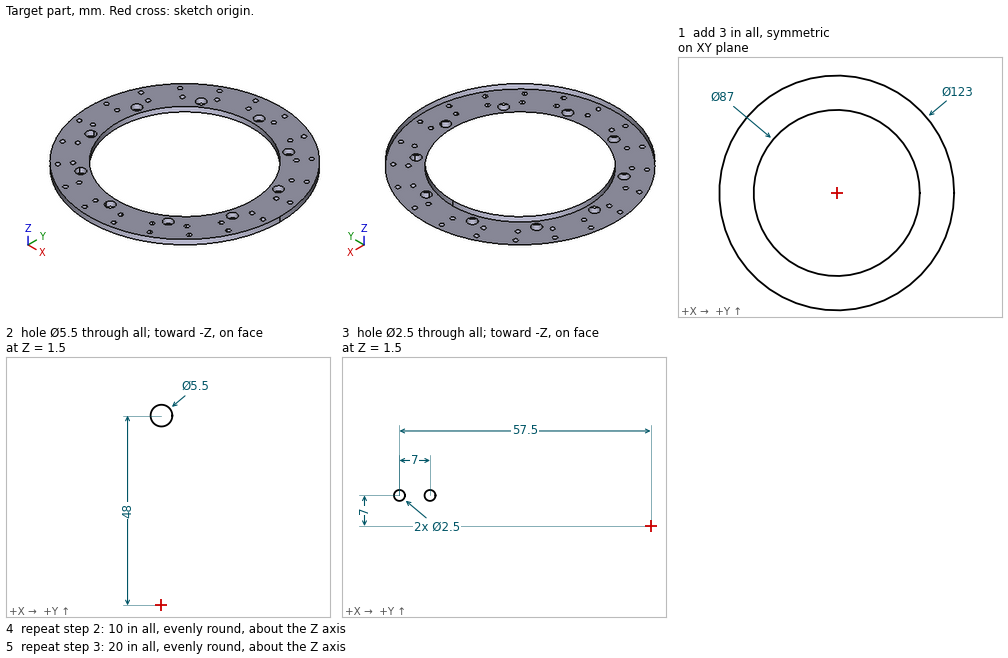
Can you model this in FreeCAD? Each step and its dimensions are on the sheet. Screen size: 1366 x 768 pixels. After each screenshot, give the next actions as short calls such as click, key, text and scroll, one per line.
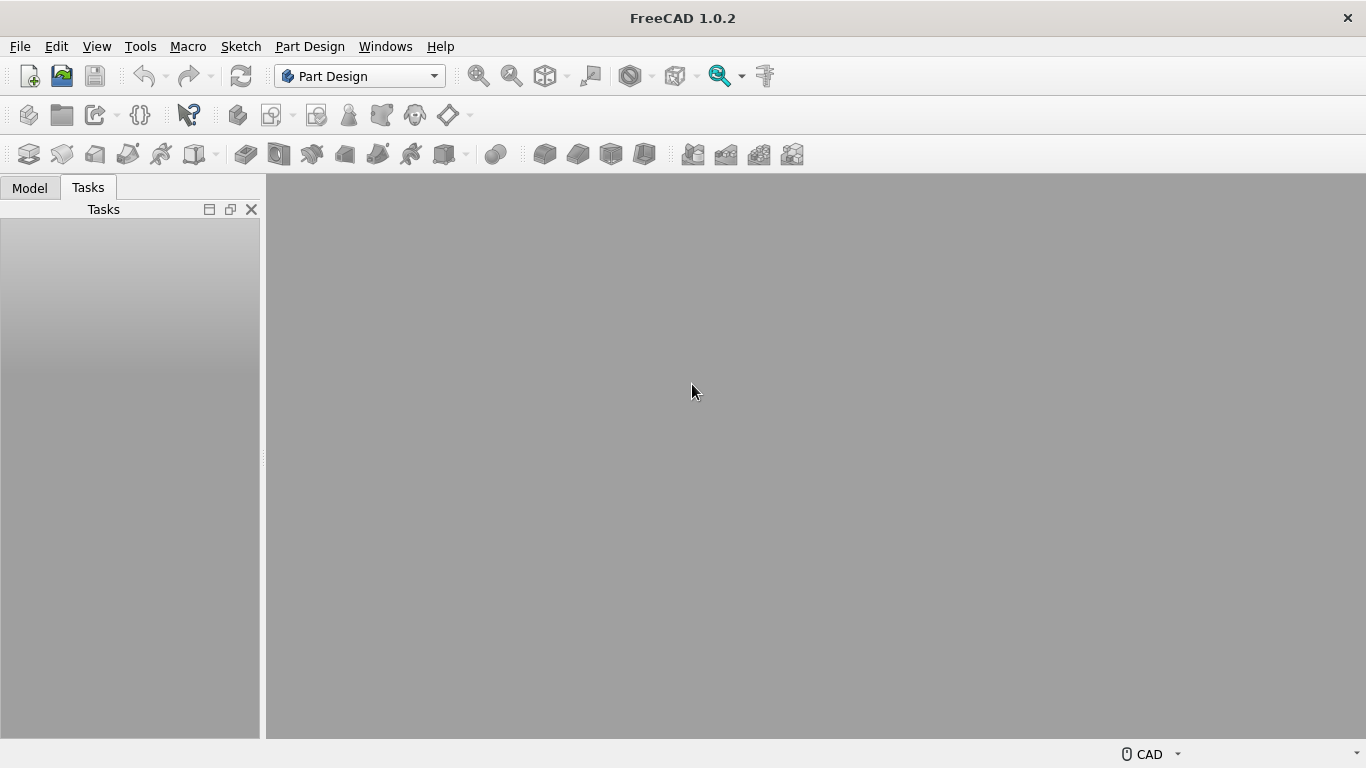
click(29, 76)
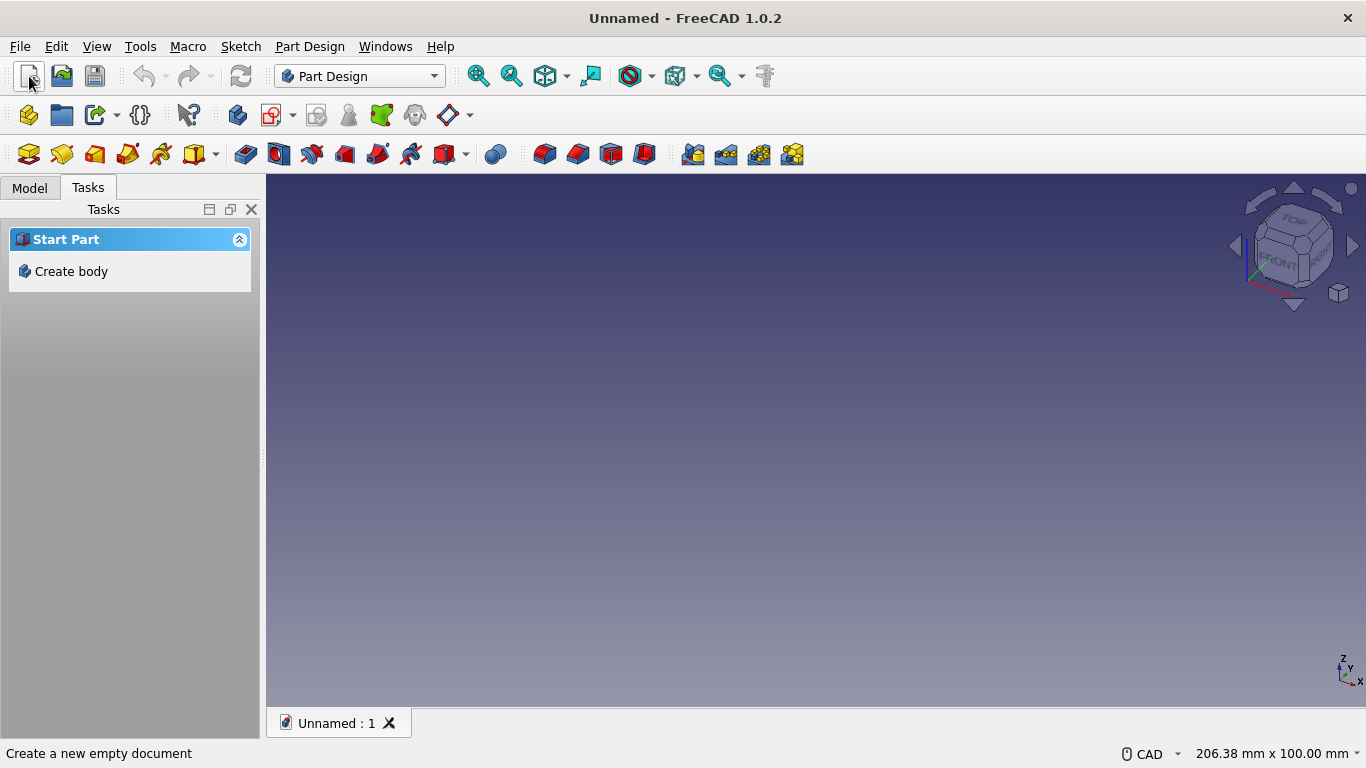
click(270, 116)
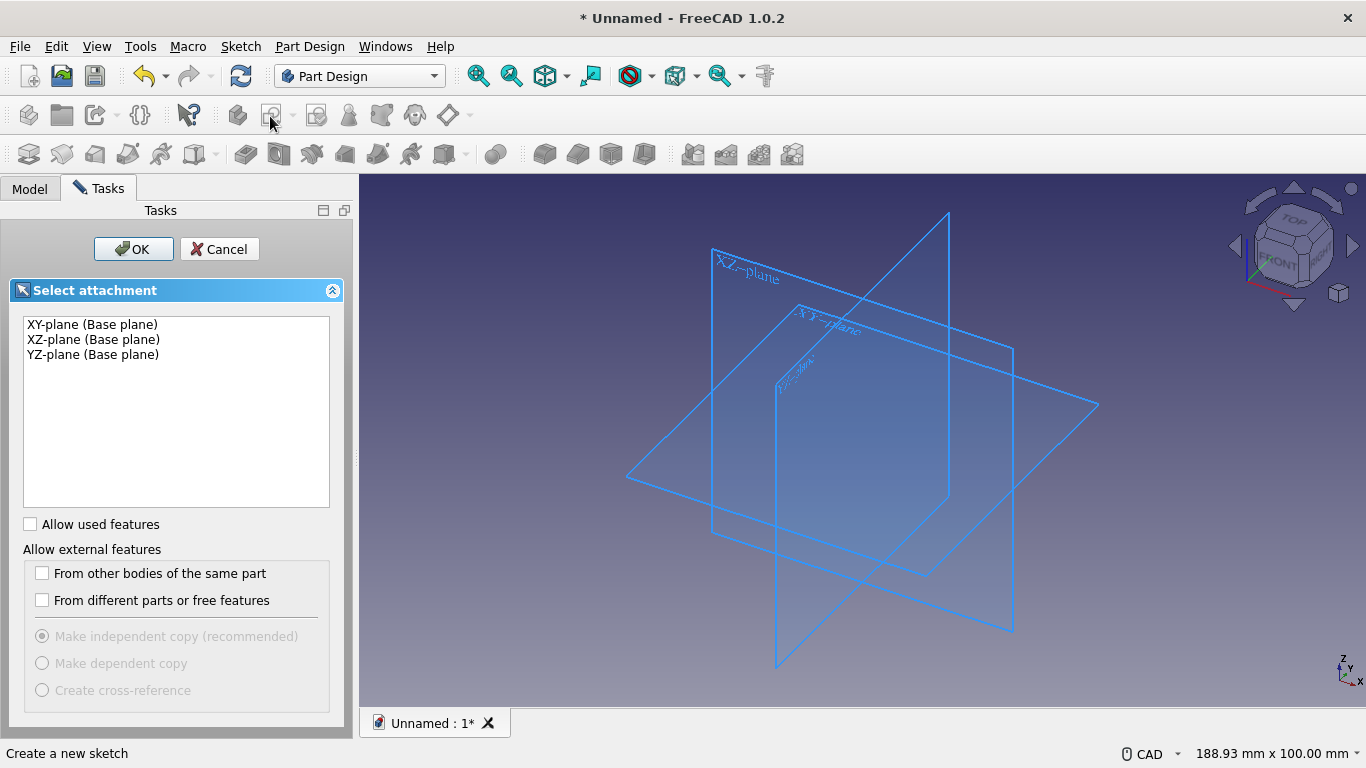
click(84, 324)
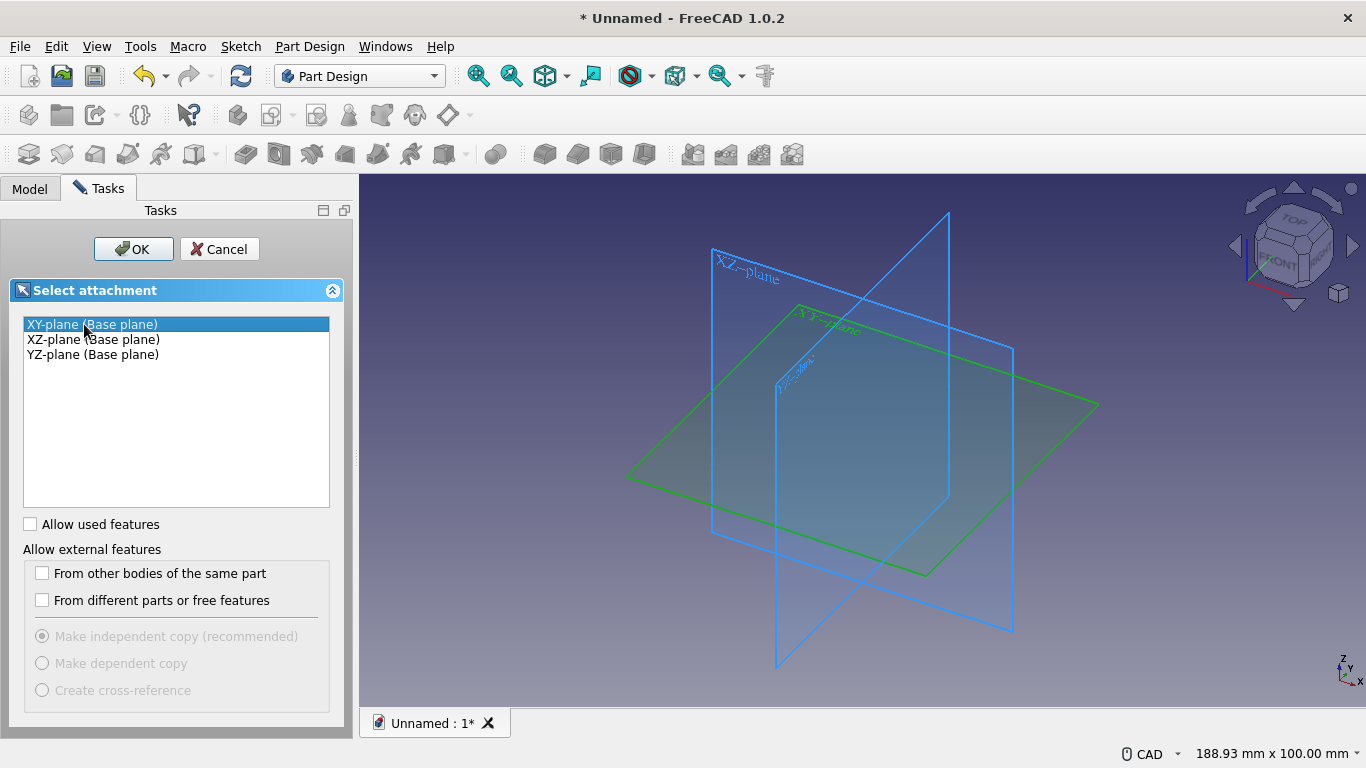
click(134, 249)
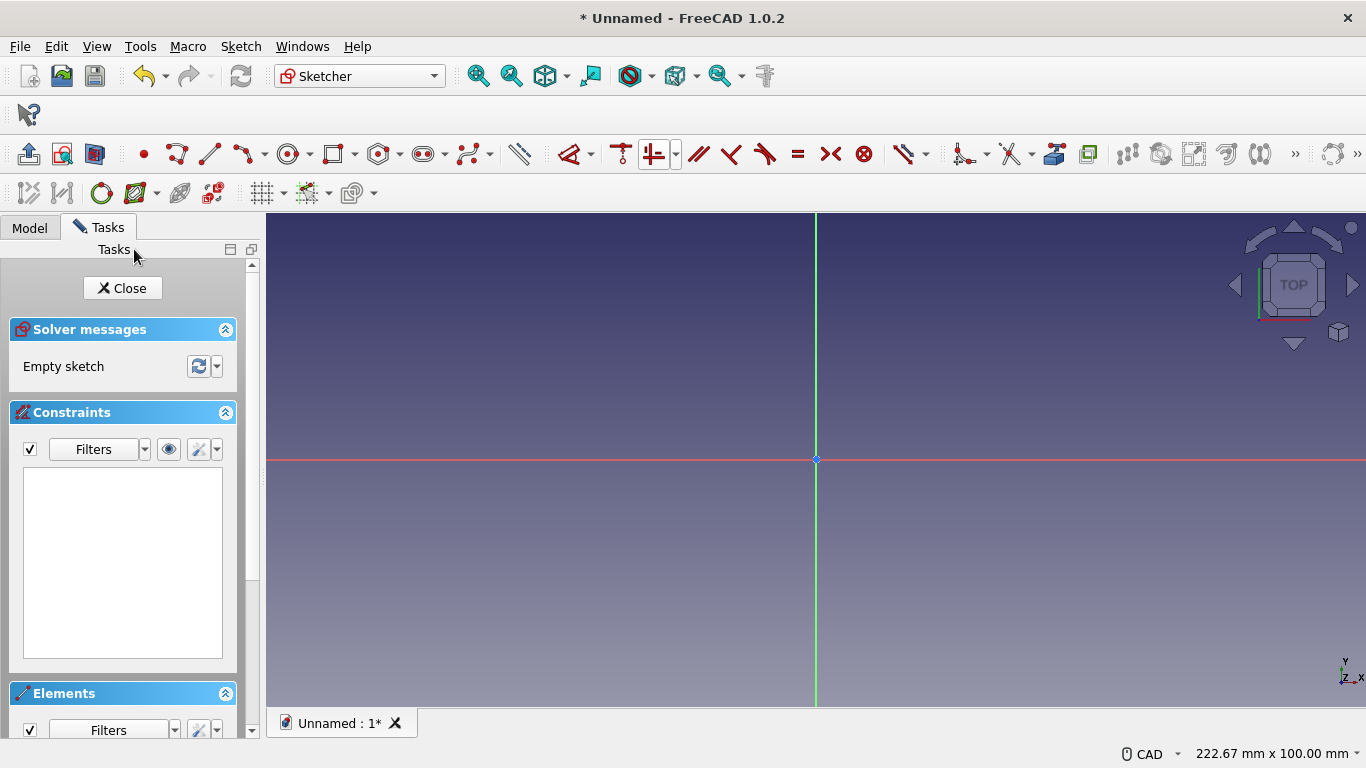
scroll(664, 460, down, 3)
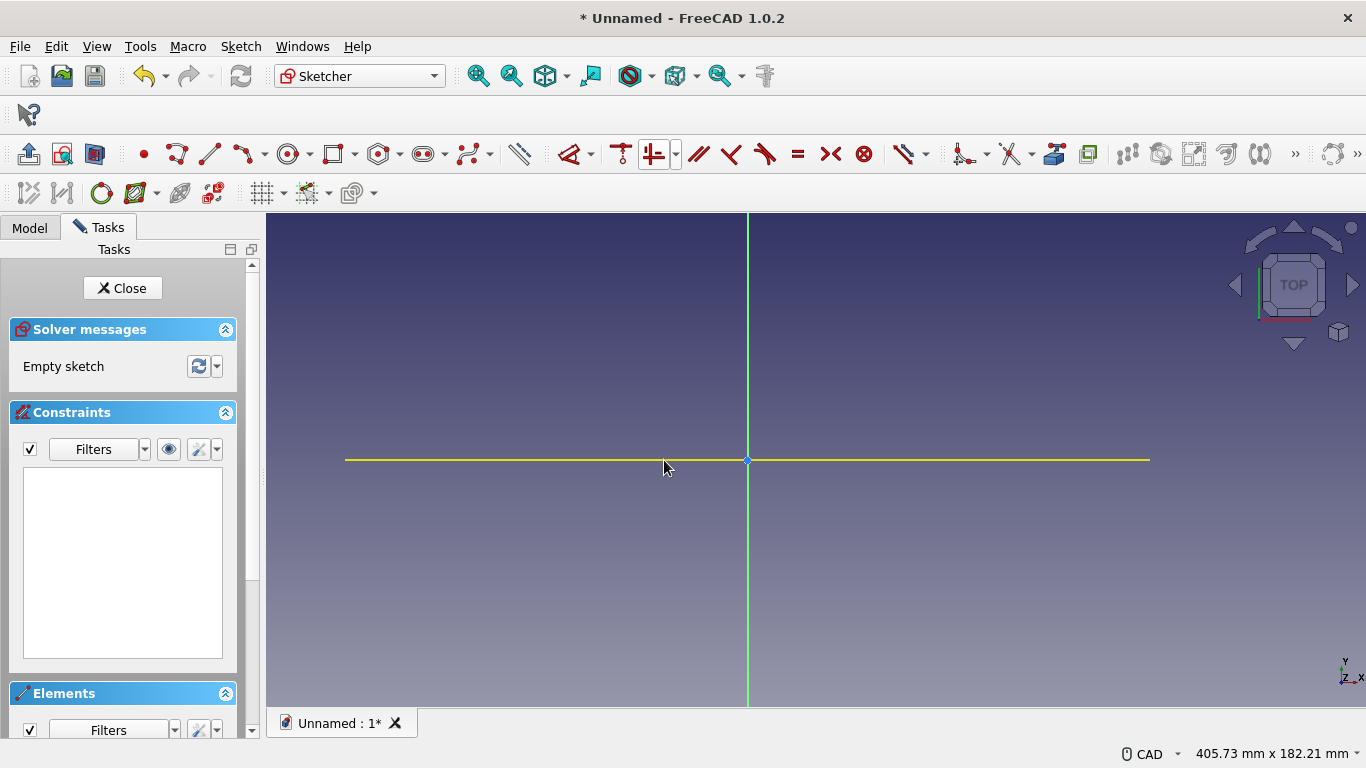
click(288, 154)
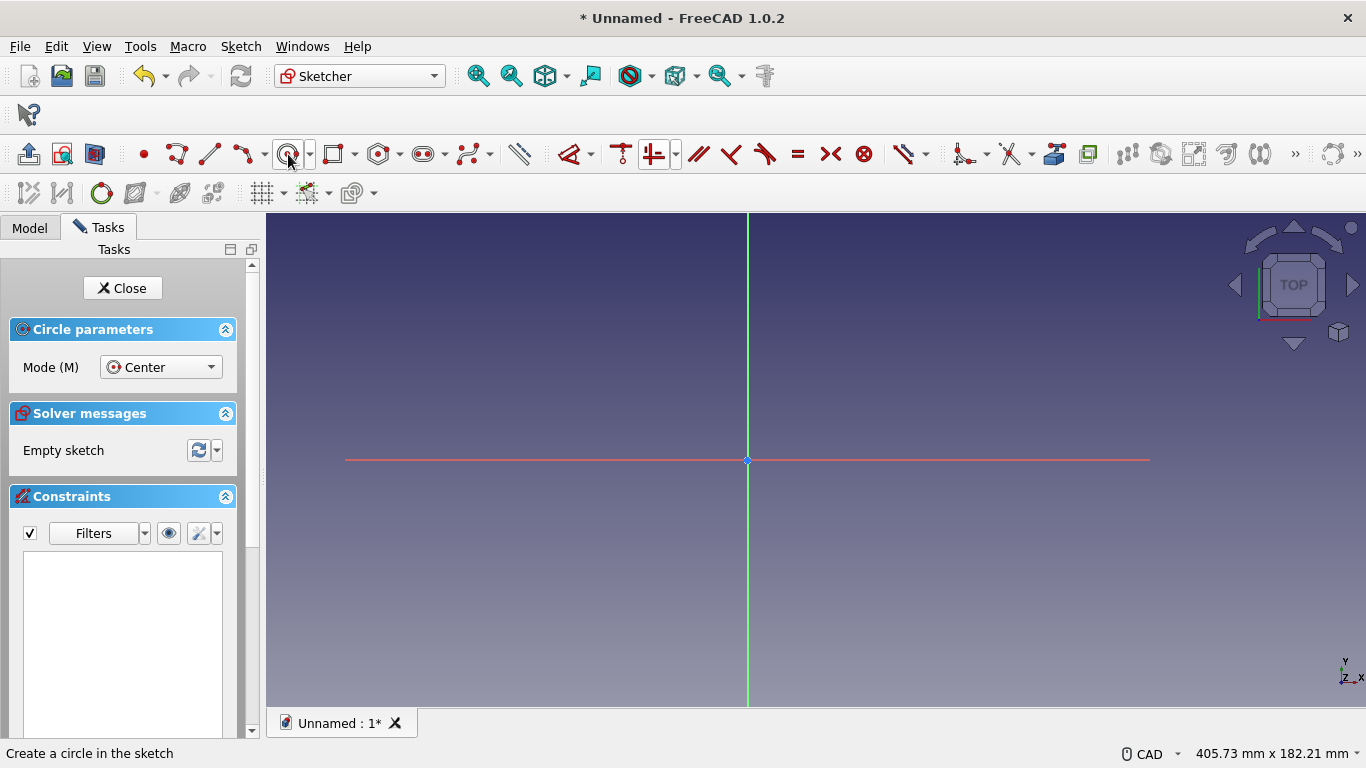
click(748, 460)
move(865, 342)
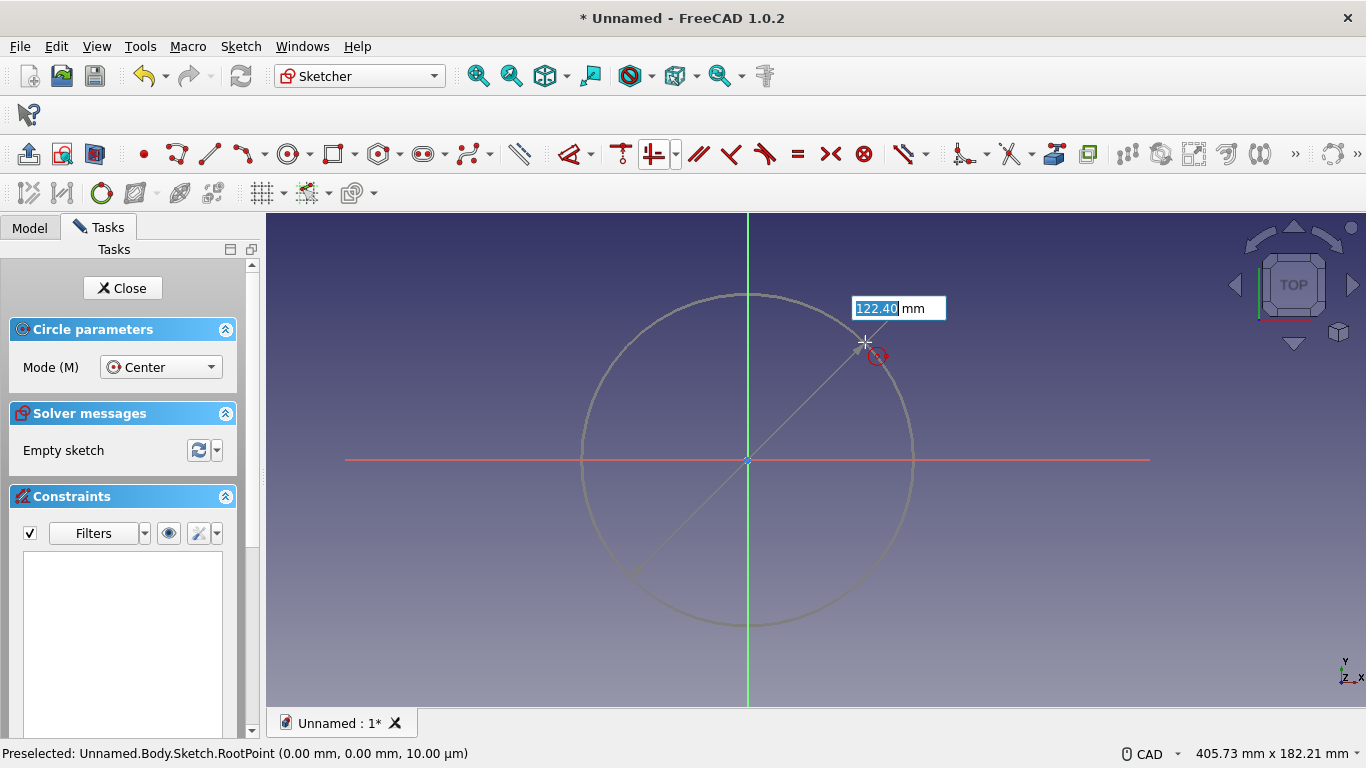
text(123)
key(Return)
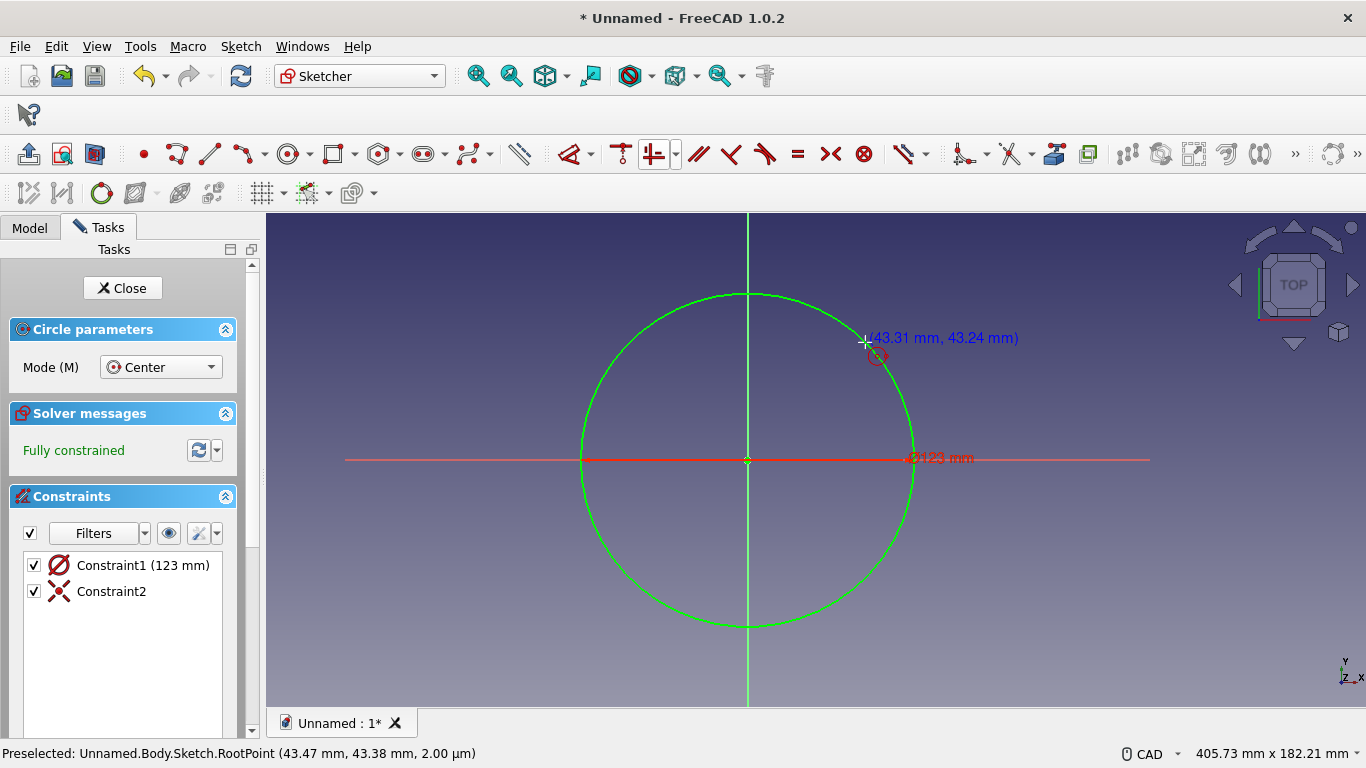
click(748, 460)
move(831, 377)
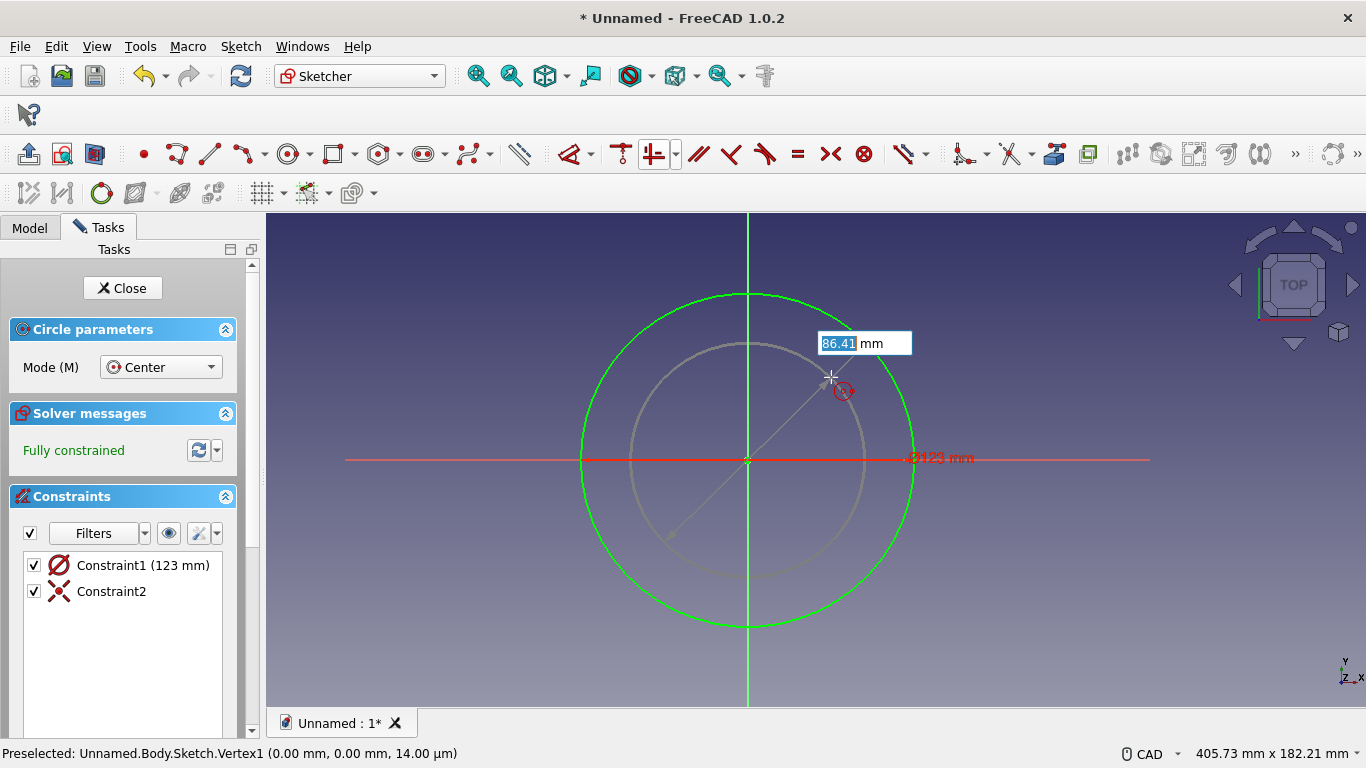
text(87)
key(Return)
key(Escape)